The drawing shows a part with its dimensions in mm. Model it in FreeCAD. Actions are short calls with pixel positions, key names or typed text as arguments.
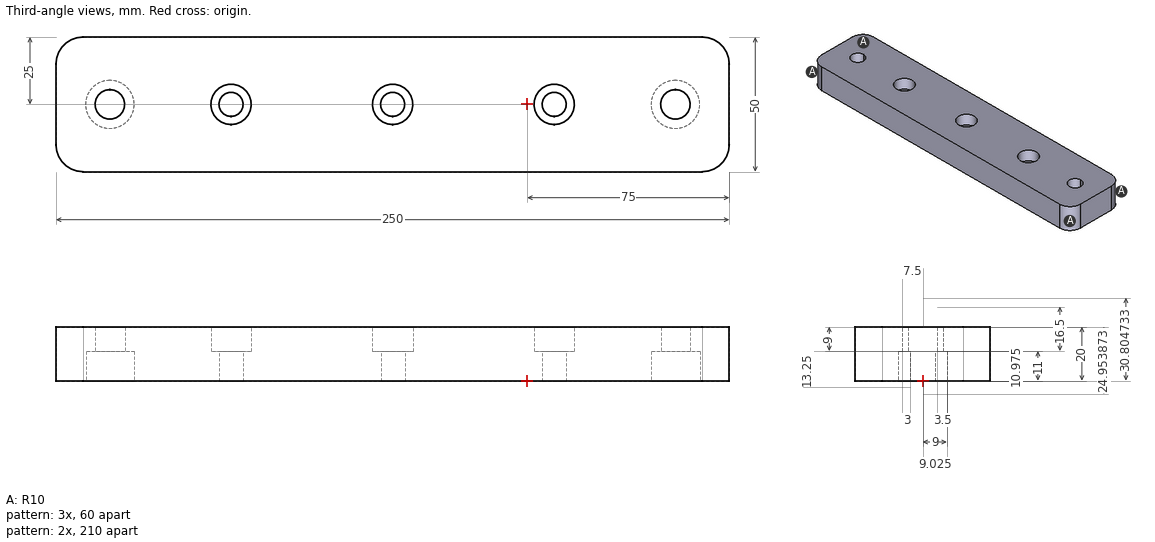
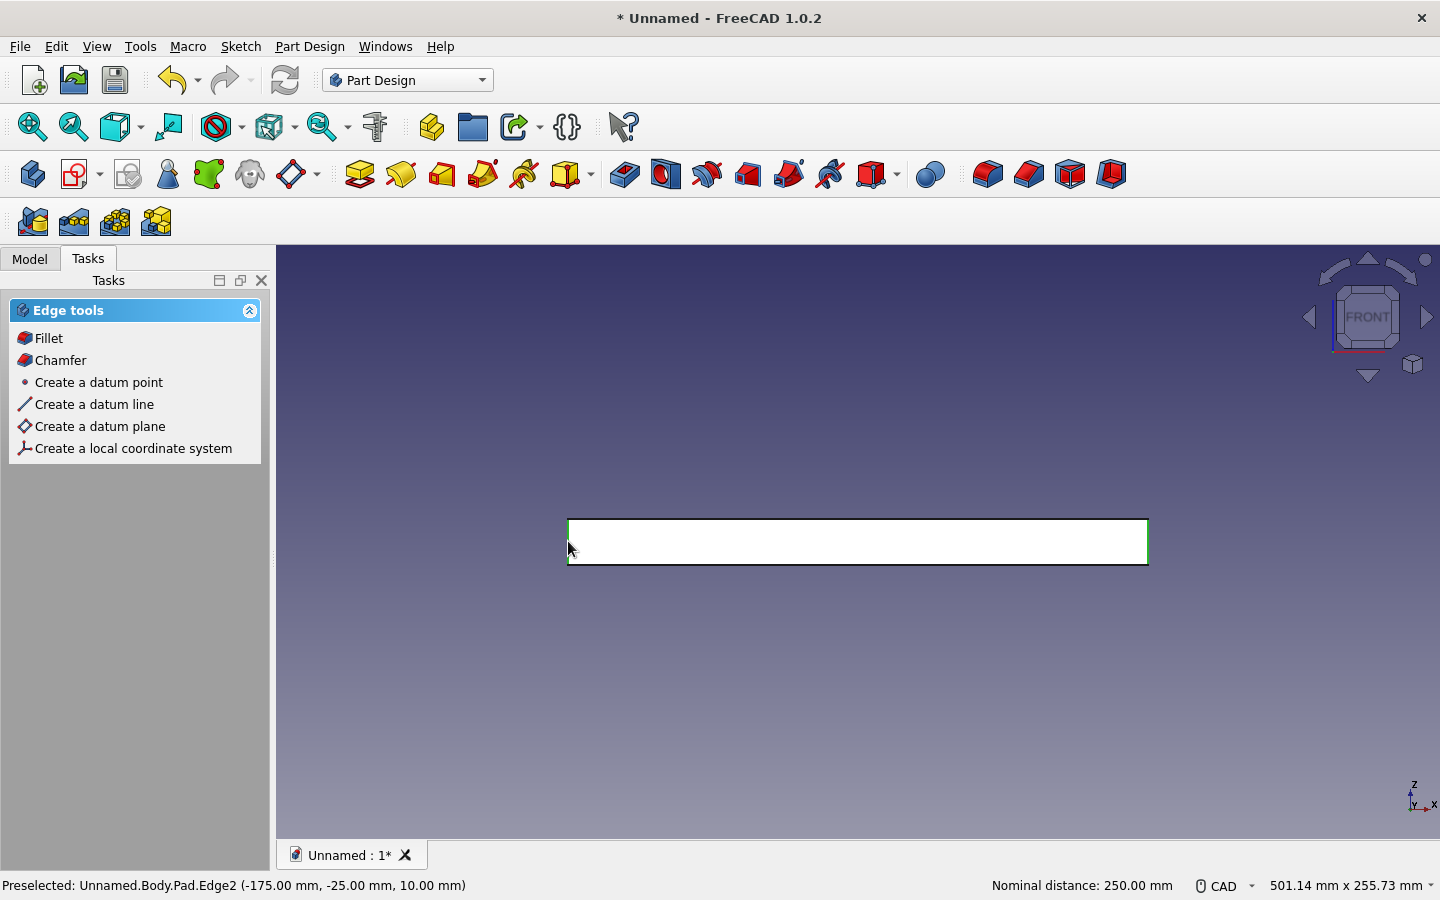
key(3)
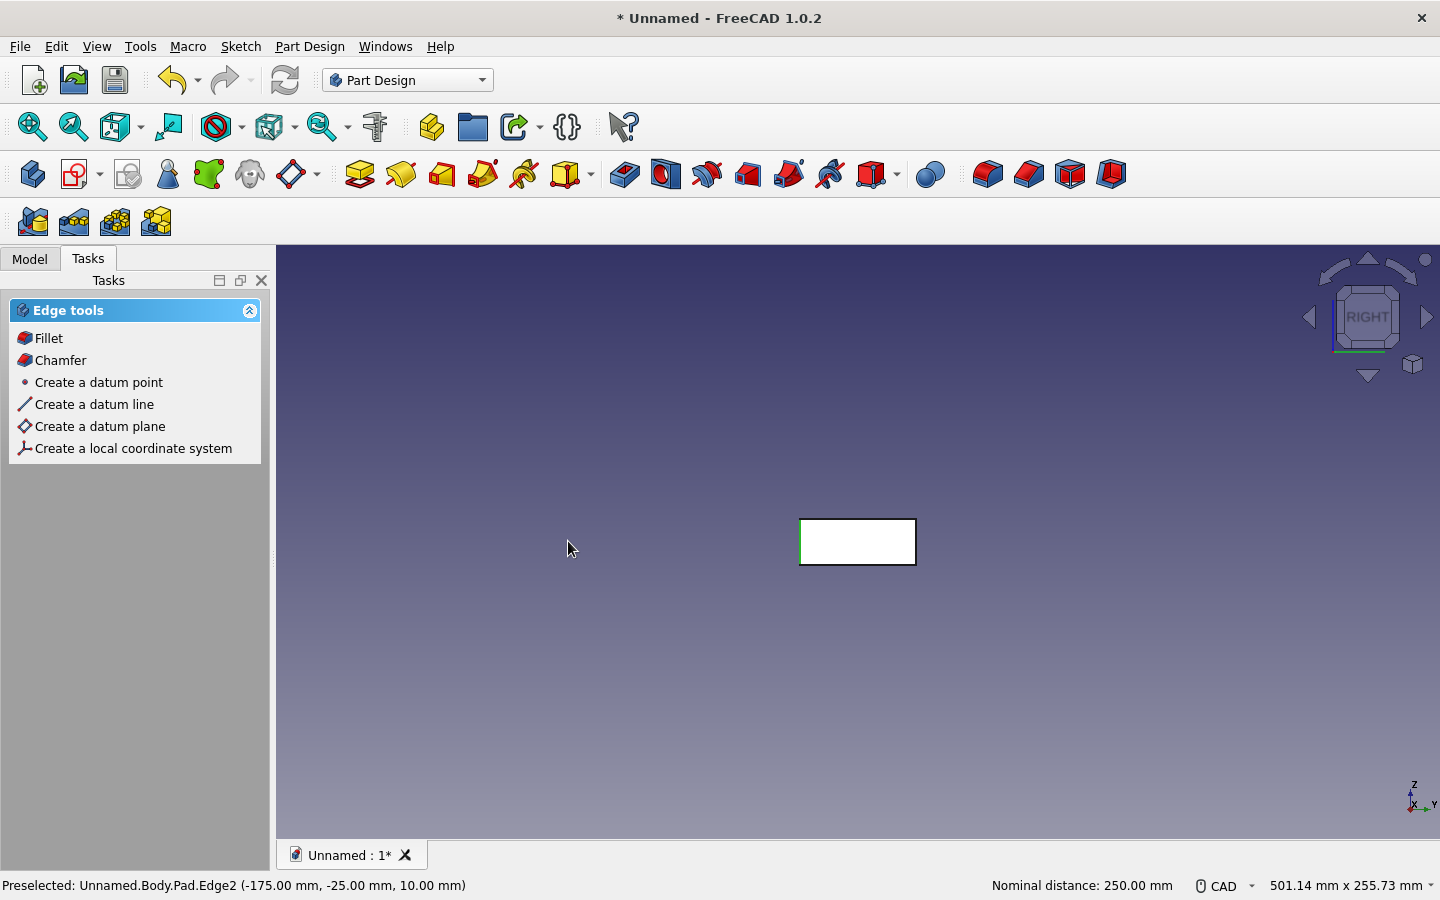
click(33, 128)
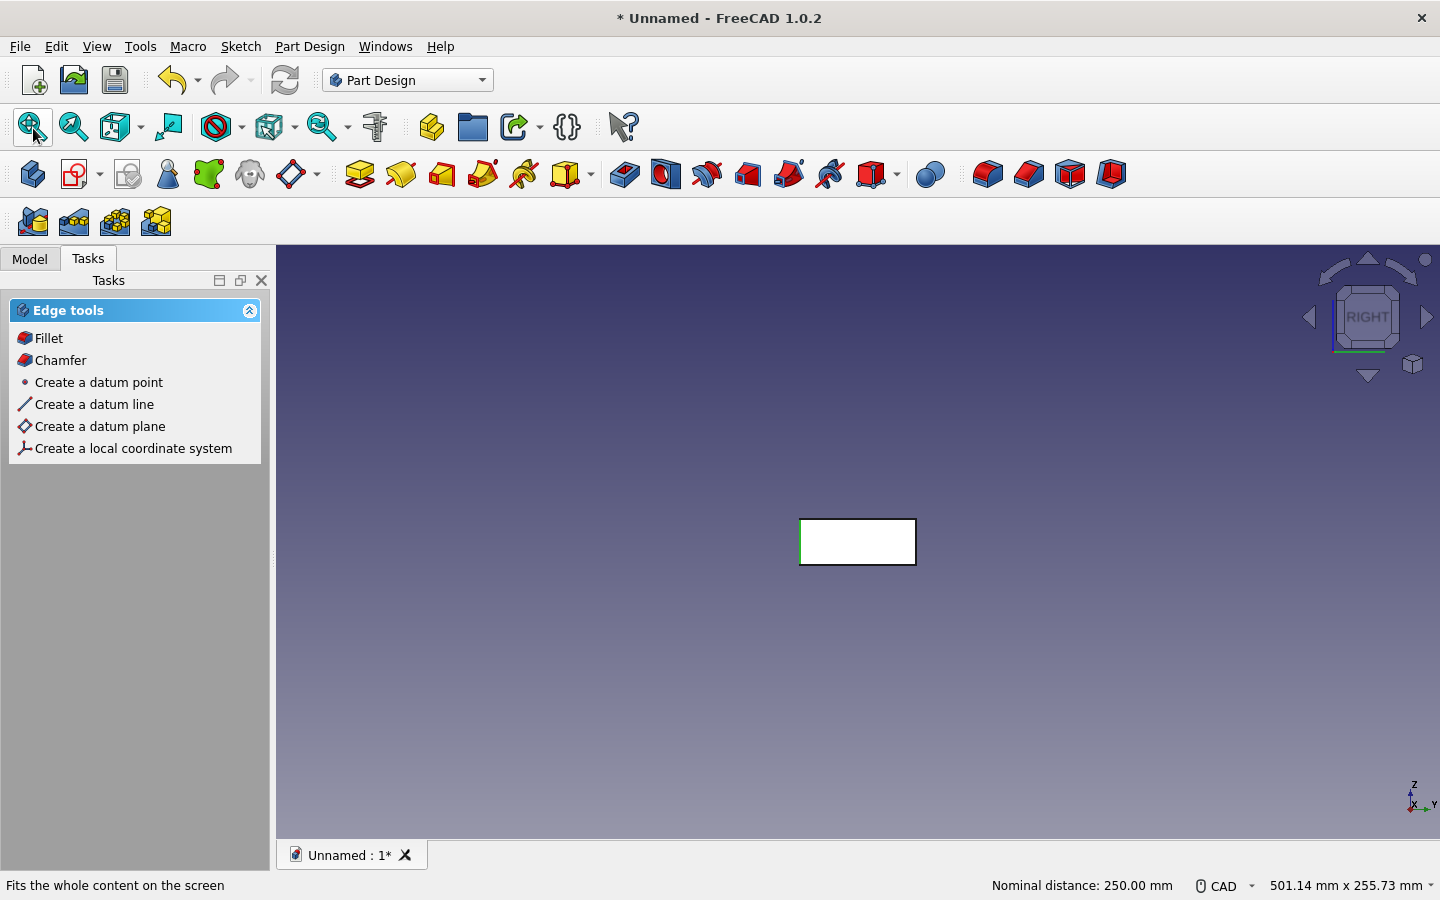
click(916, 541, ctrl)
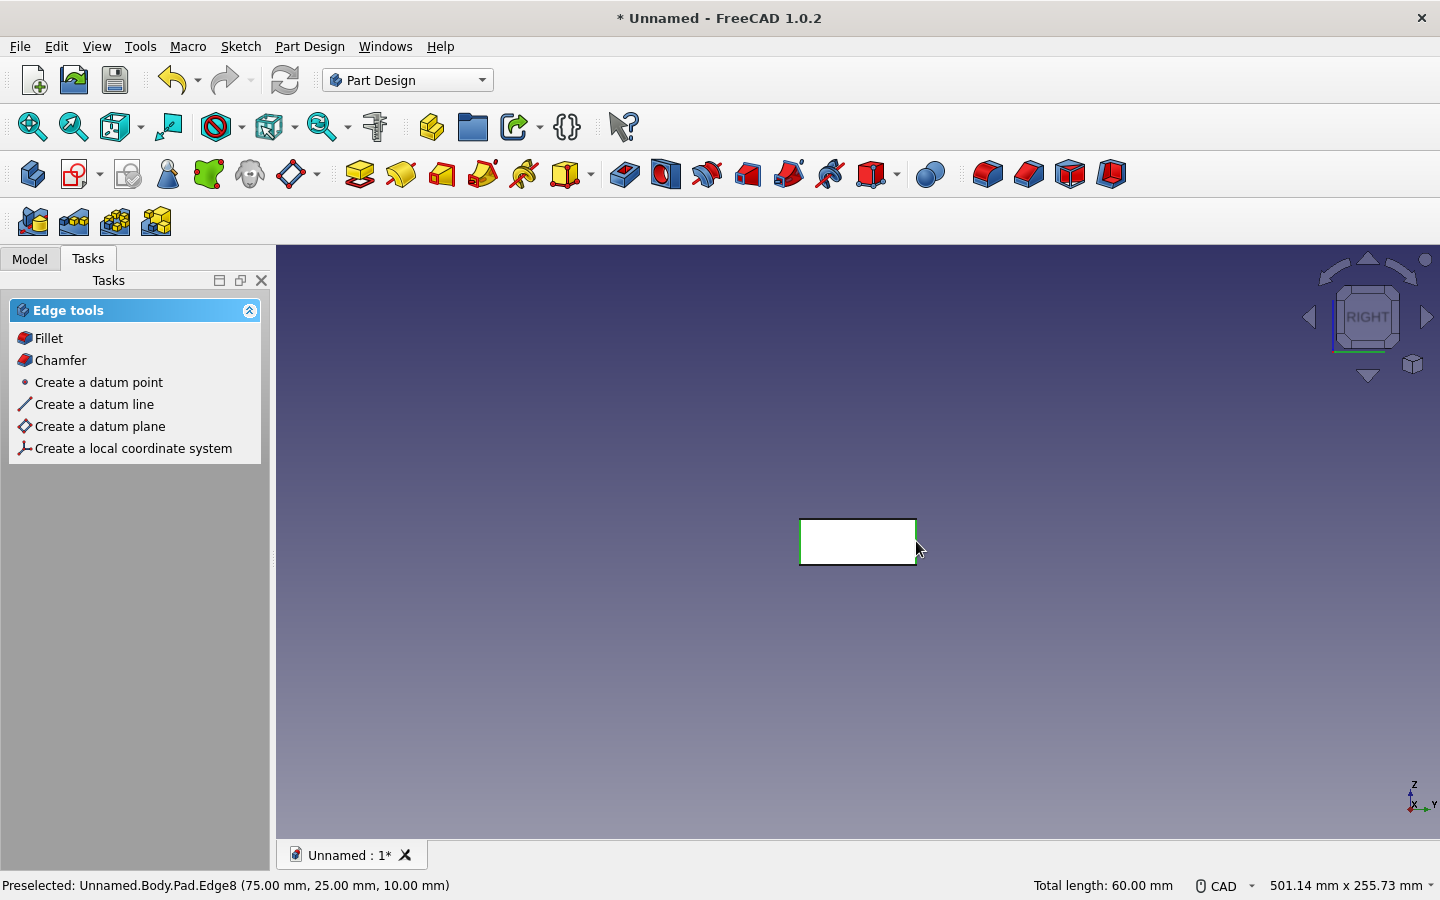
key(5)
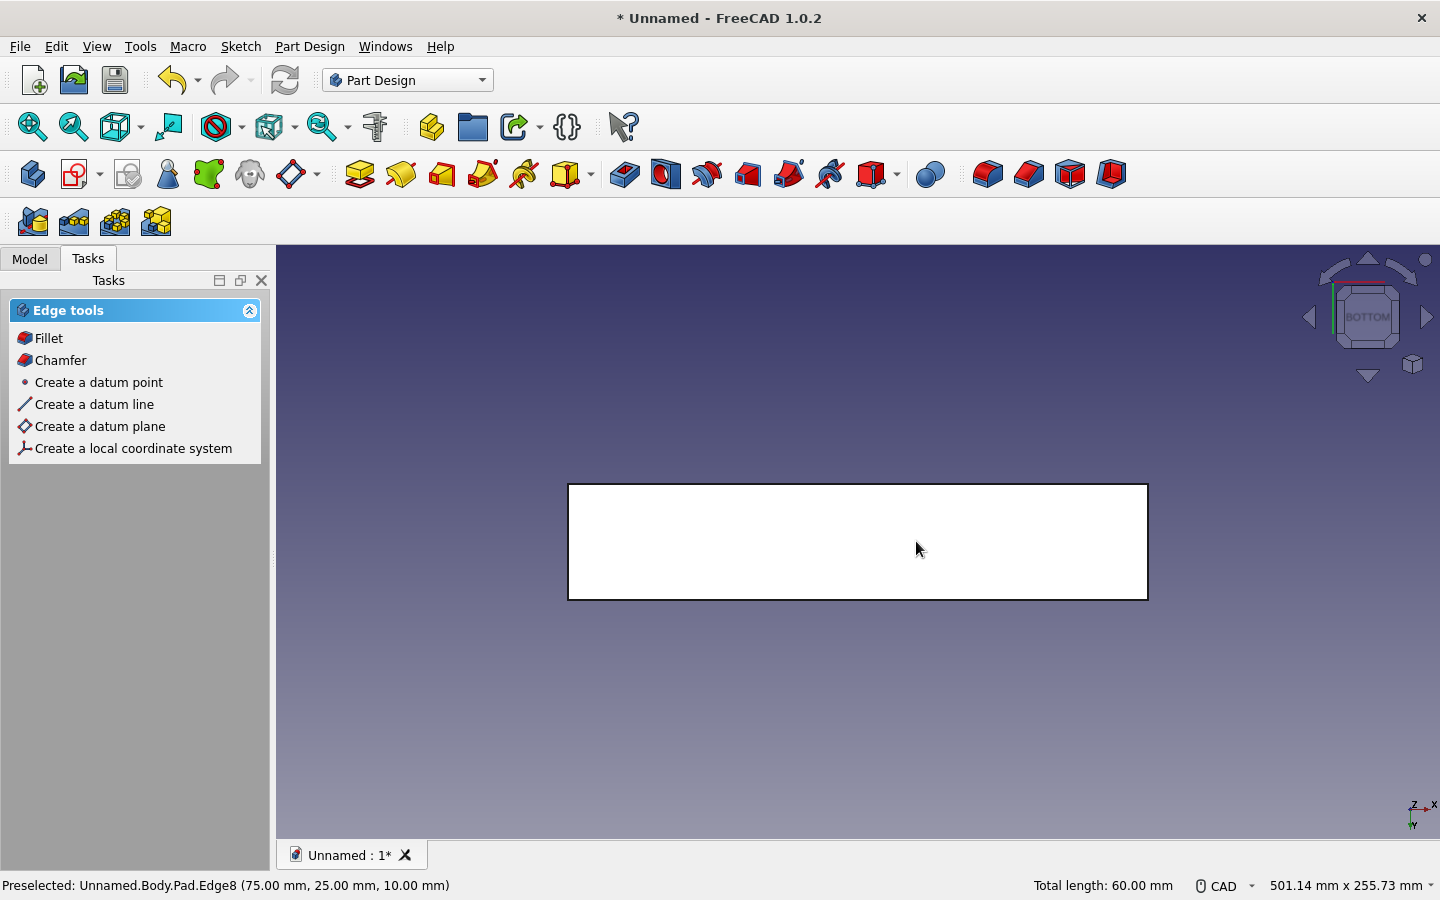
key(4)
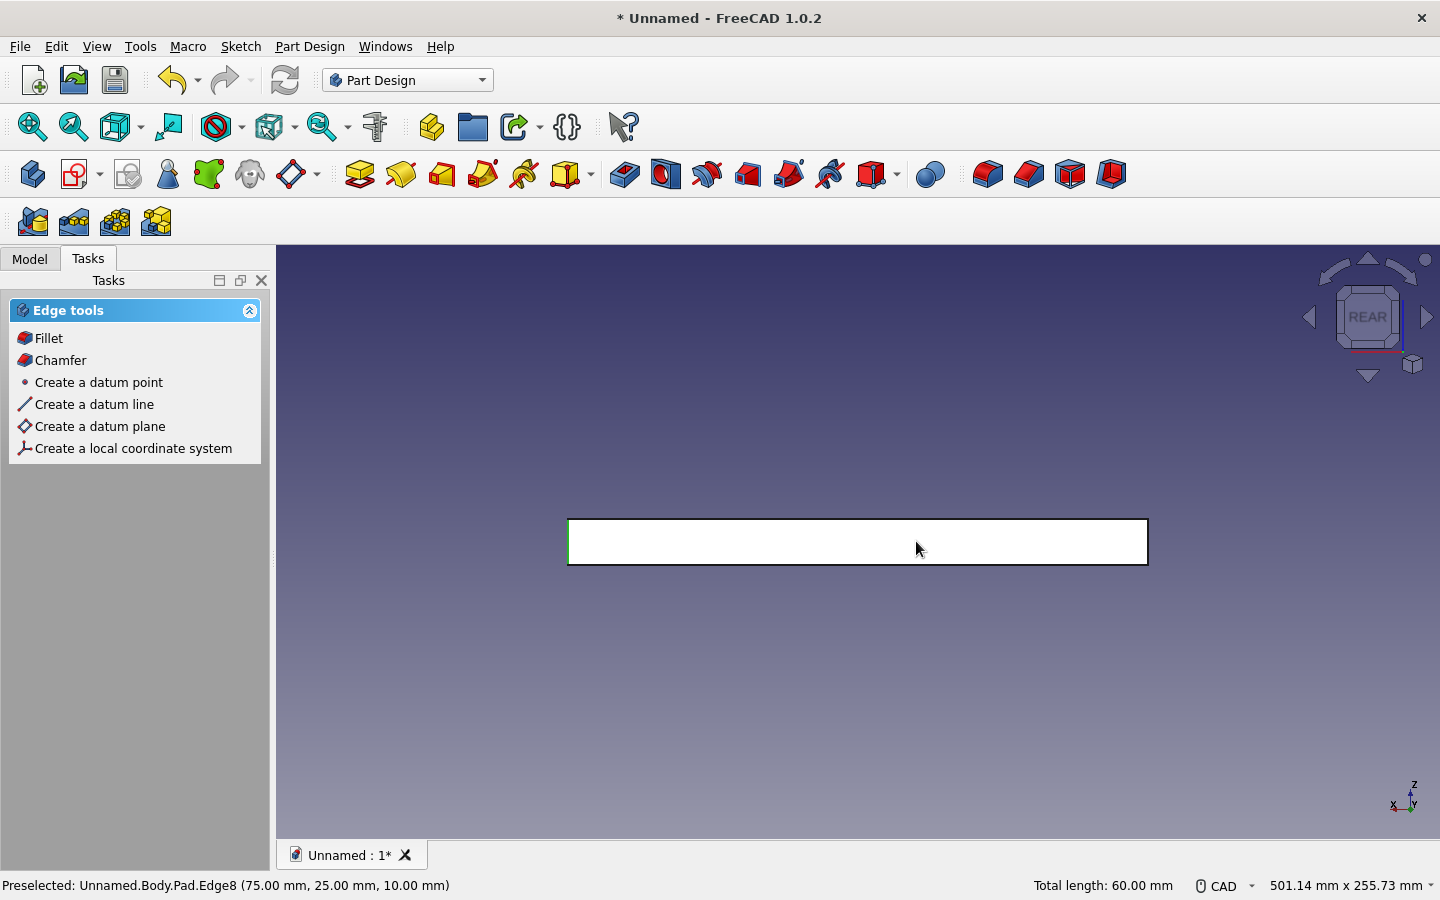
click(1148, 541, ctrl)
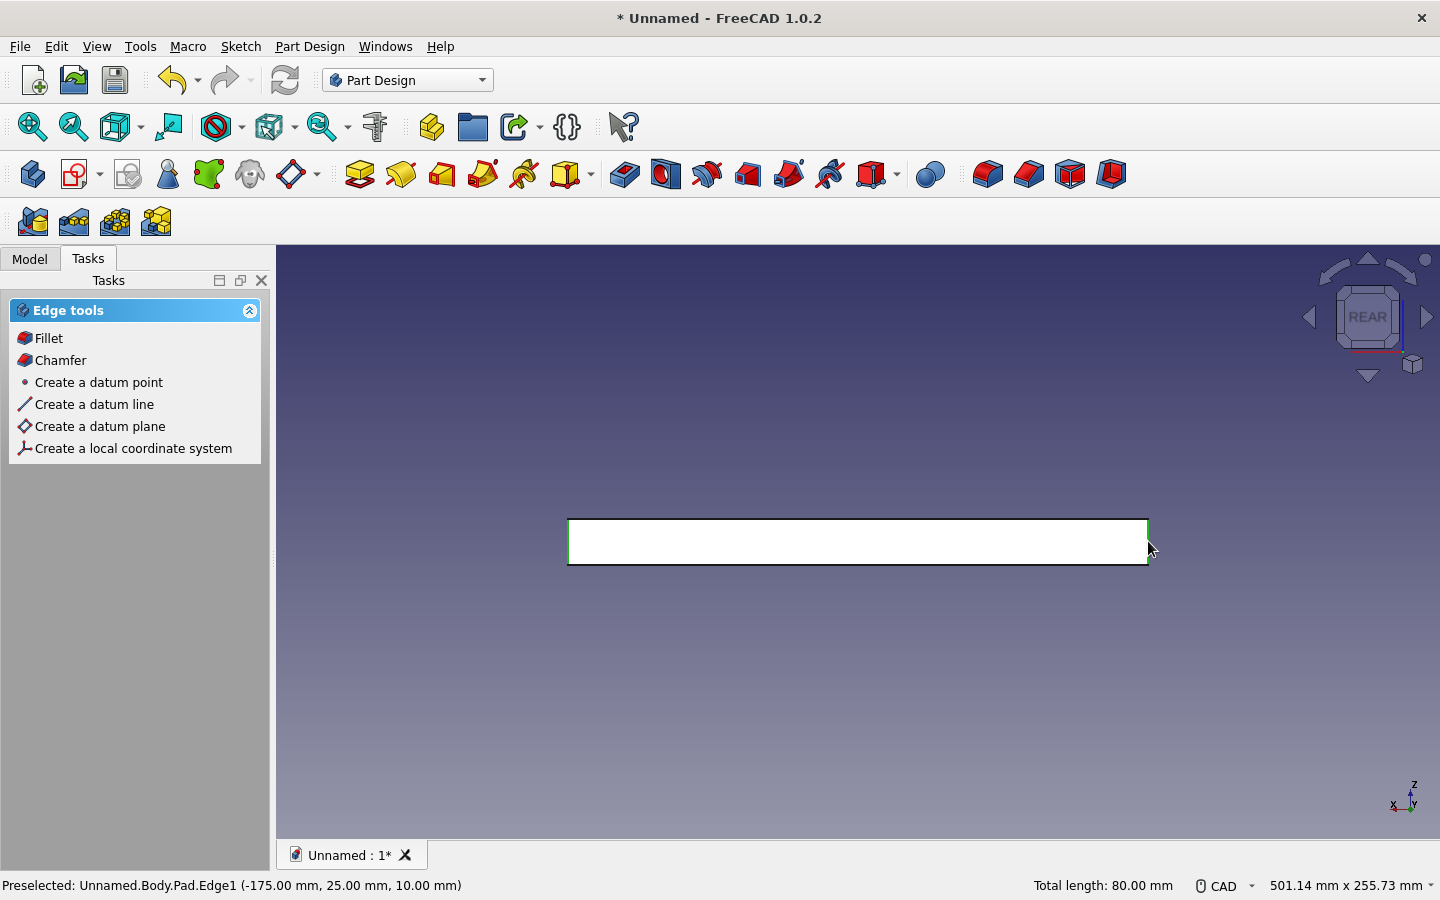
click(988, 174)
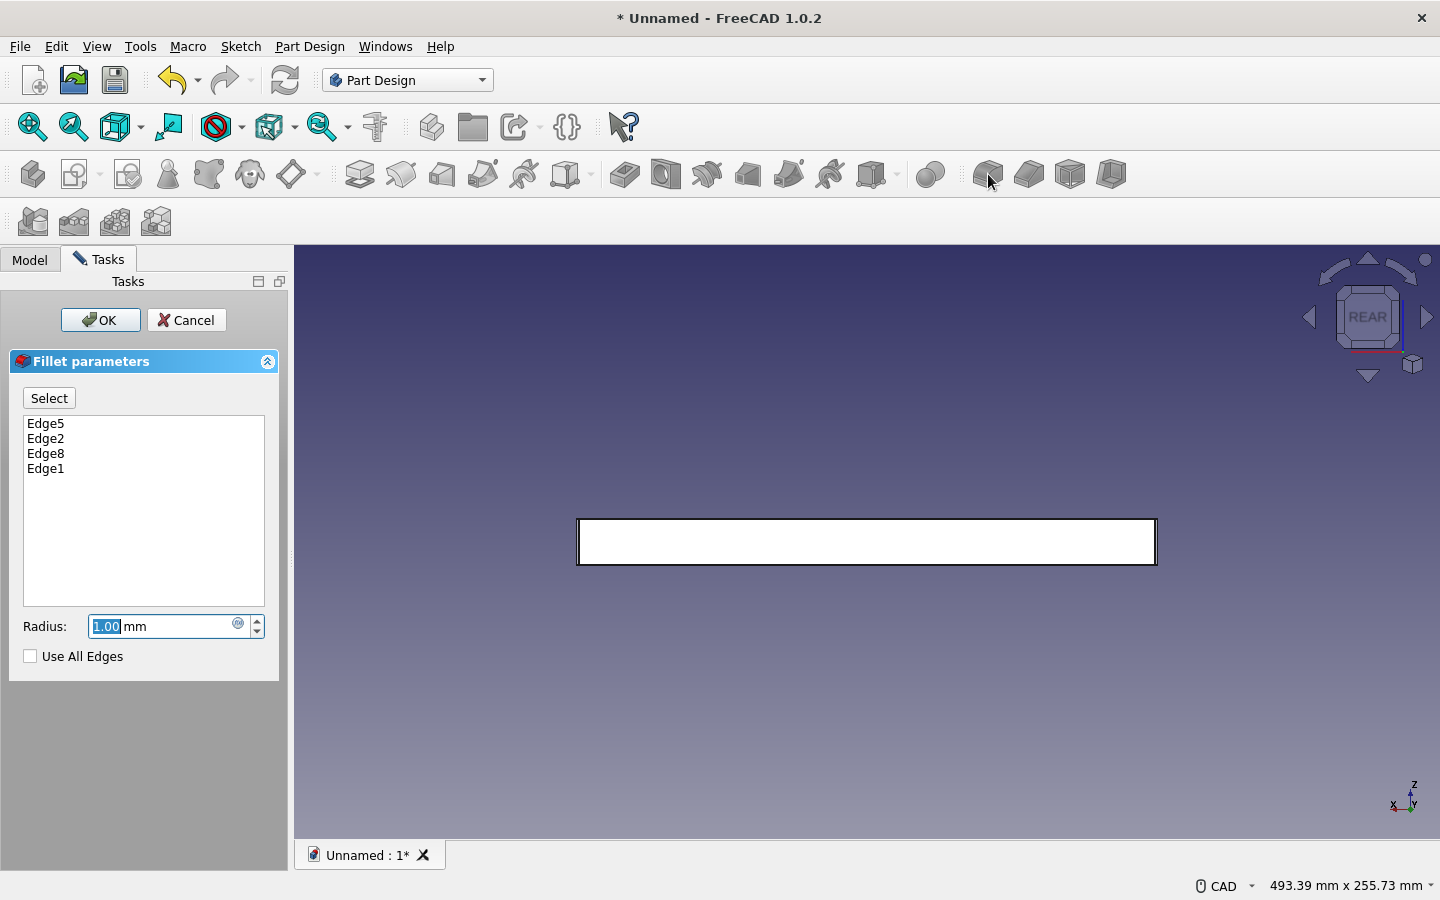
text(10)
key(Tab)